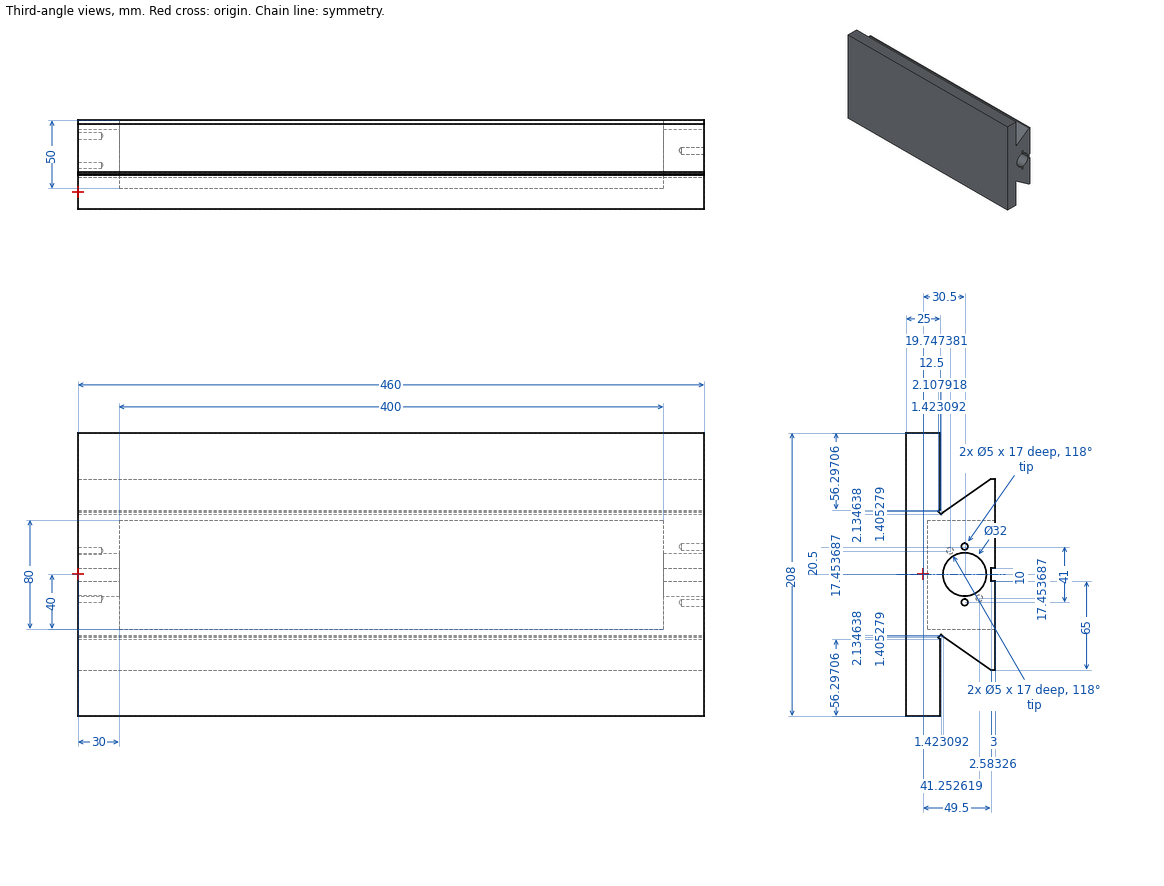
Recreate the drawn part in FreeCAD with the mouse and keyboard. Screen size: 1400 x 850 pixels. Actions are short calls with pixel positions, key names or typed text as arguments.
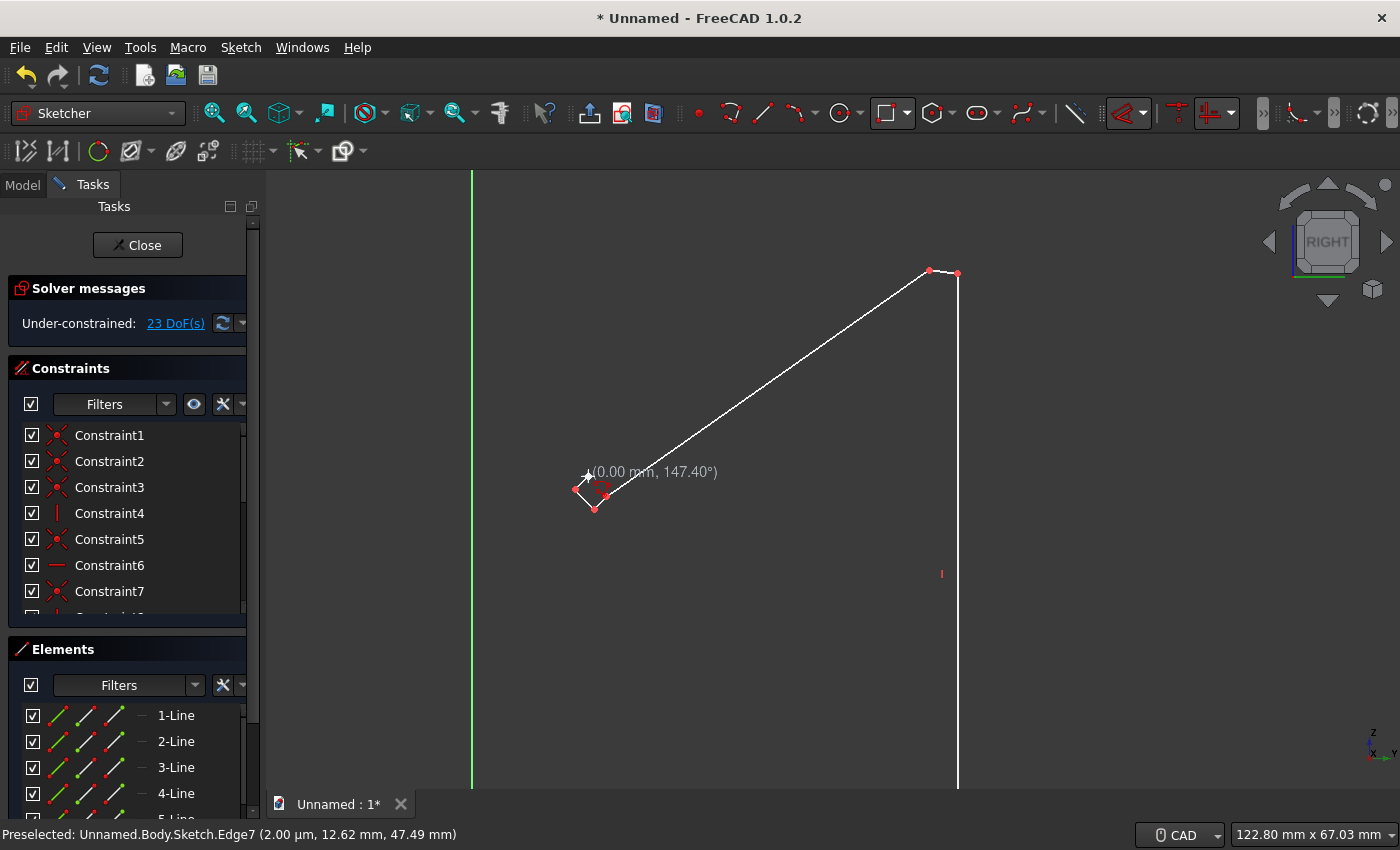
scroll(792, 369, down, 8)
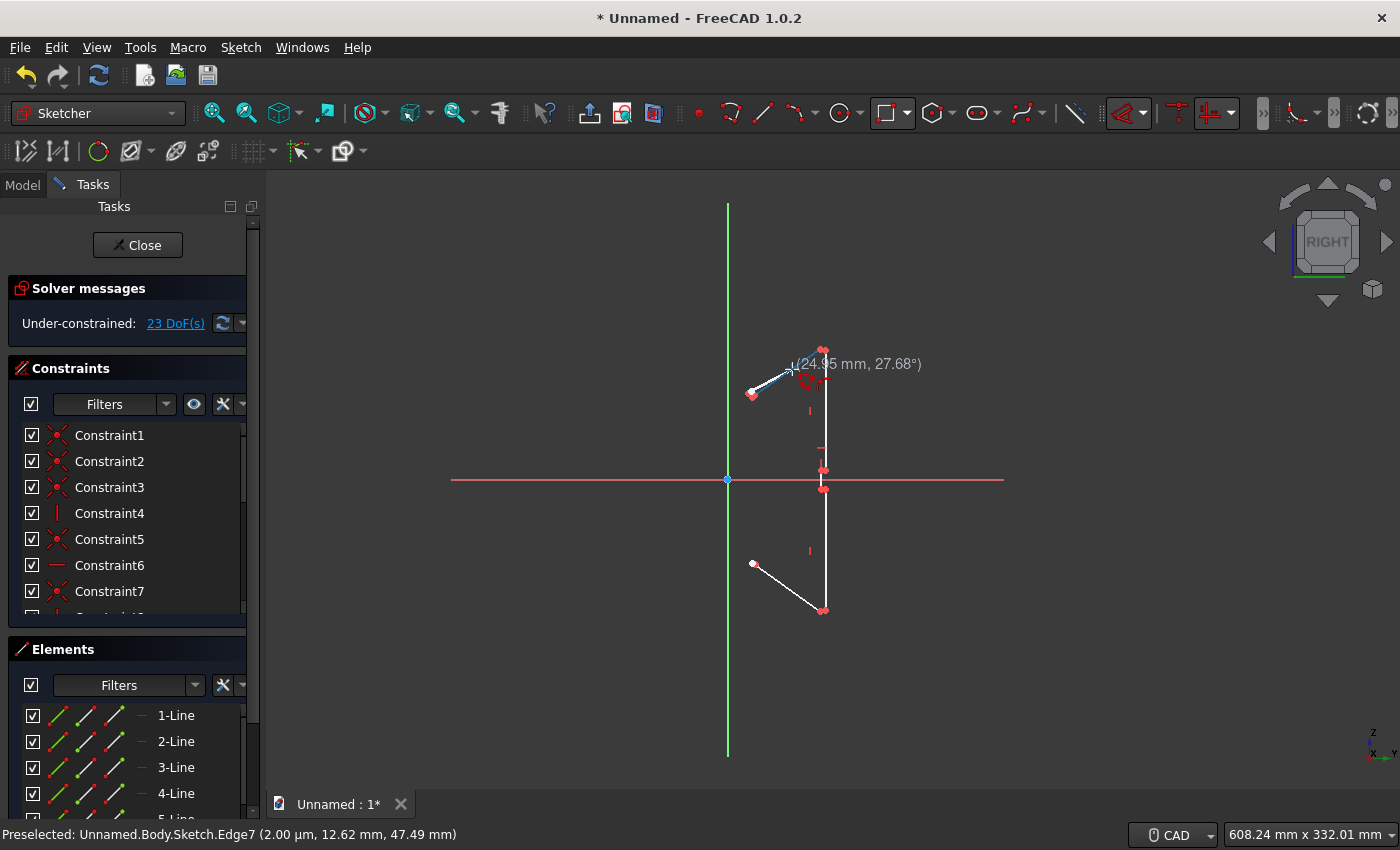
click(751, 286)
click(705, 286)
click(705, 674)
click(751, 674)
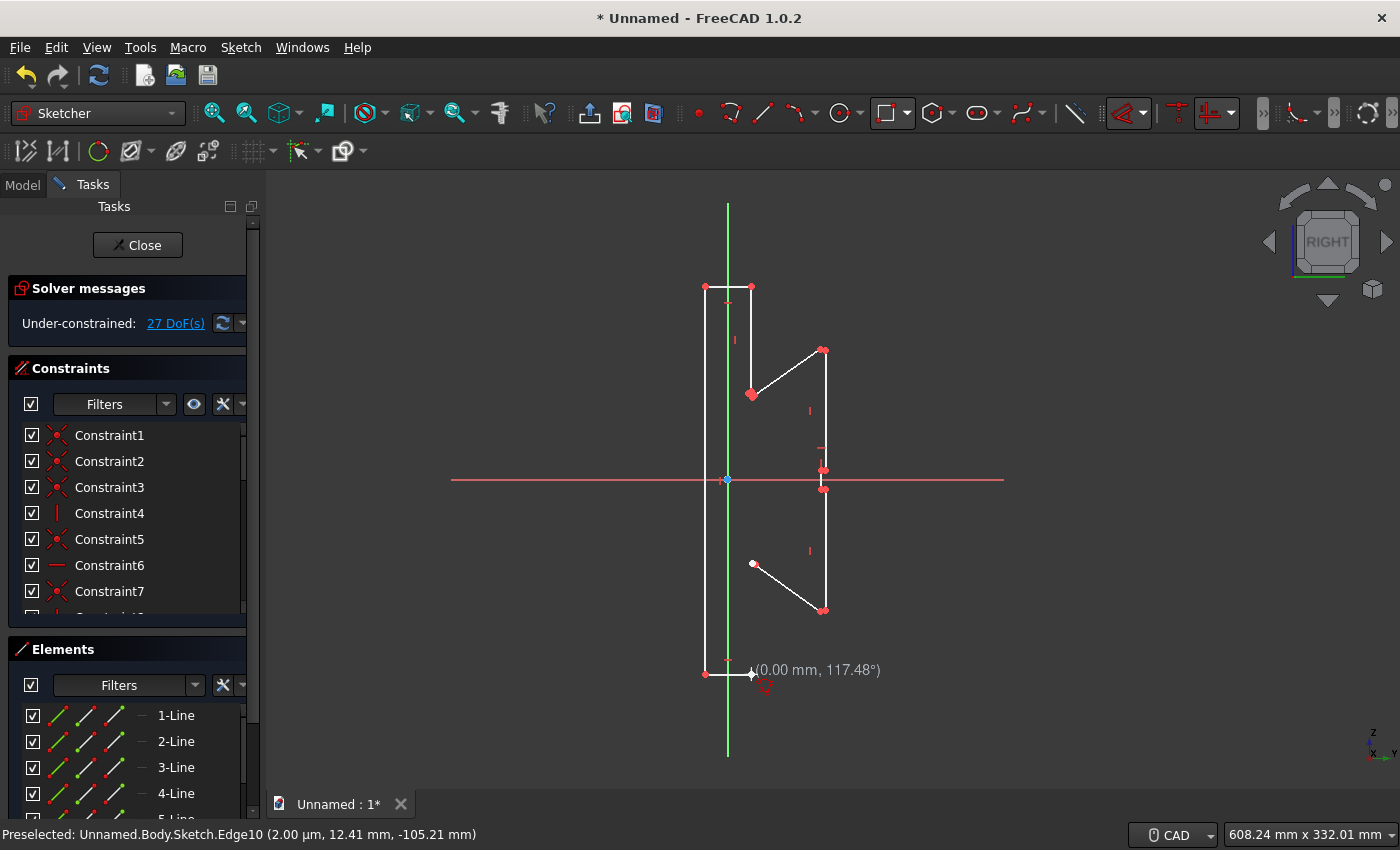
scroll(751, 569, up, 6)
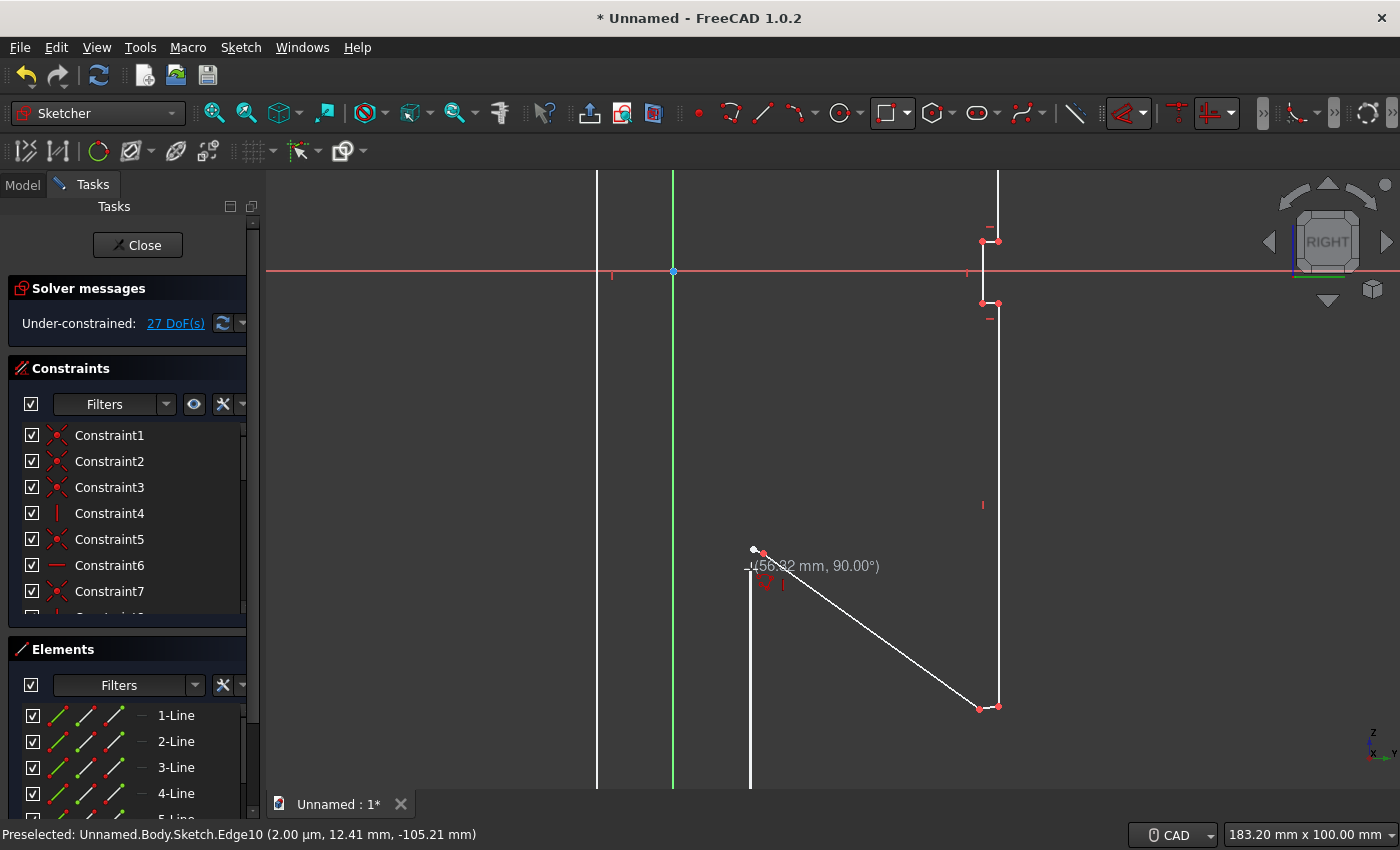
click(750, 567)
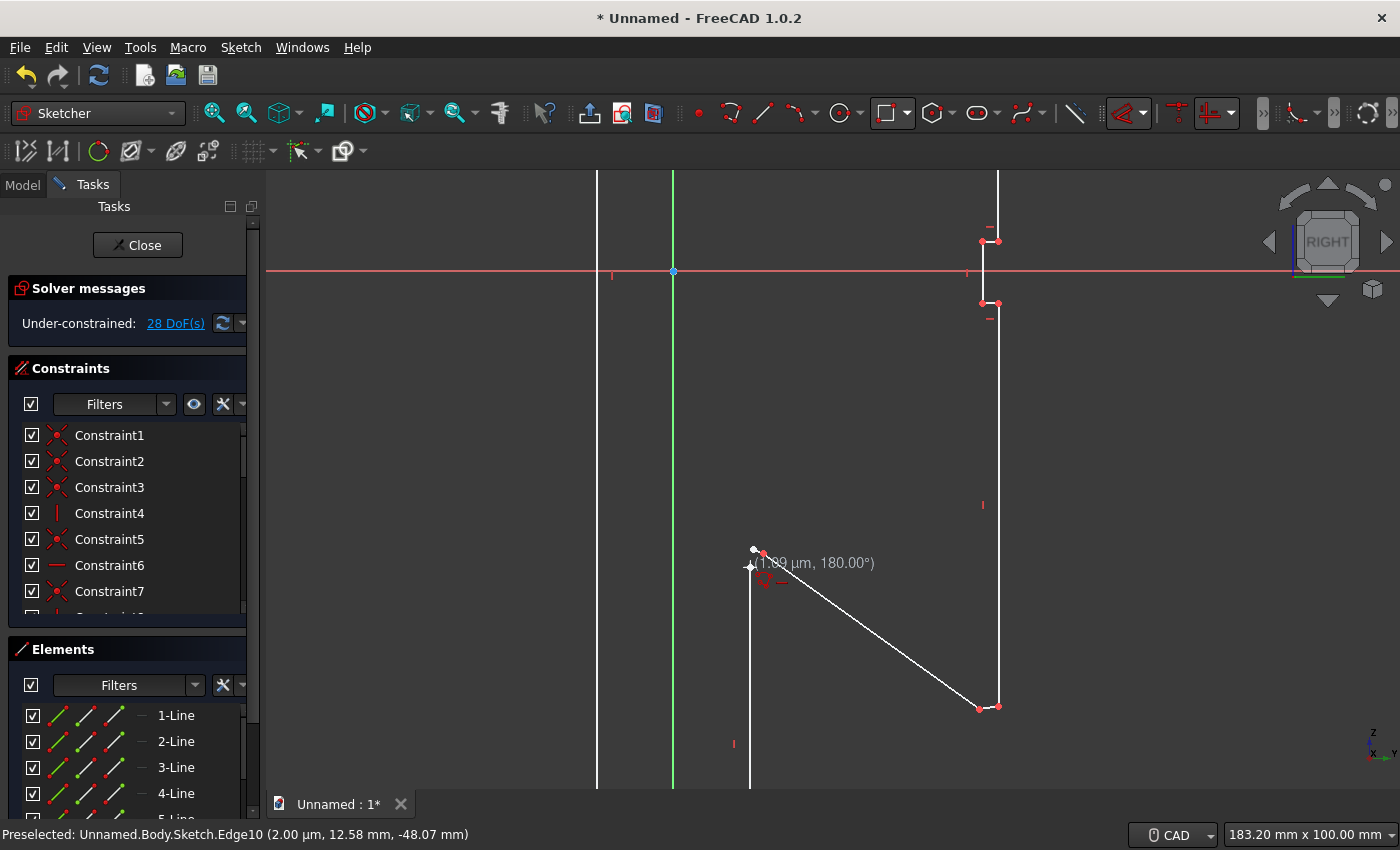
scroll(742, 558, up, 2)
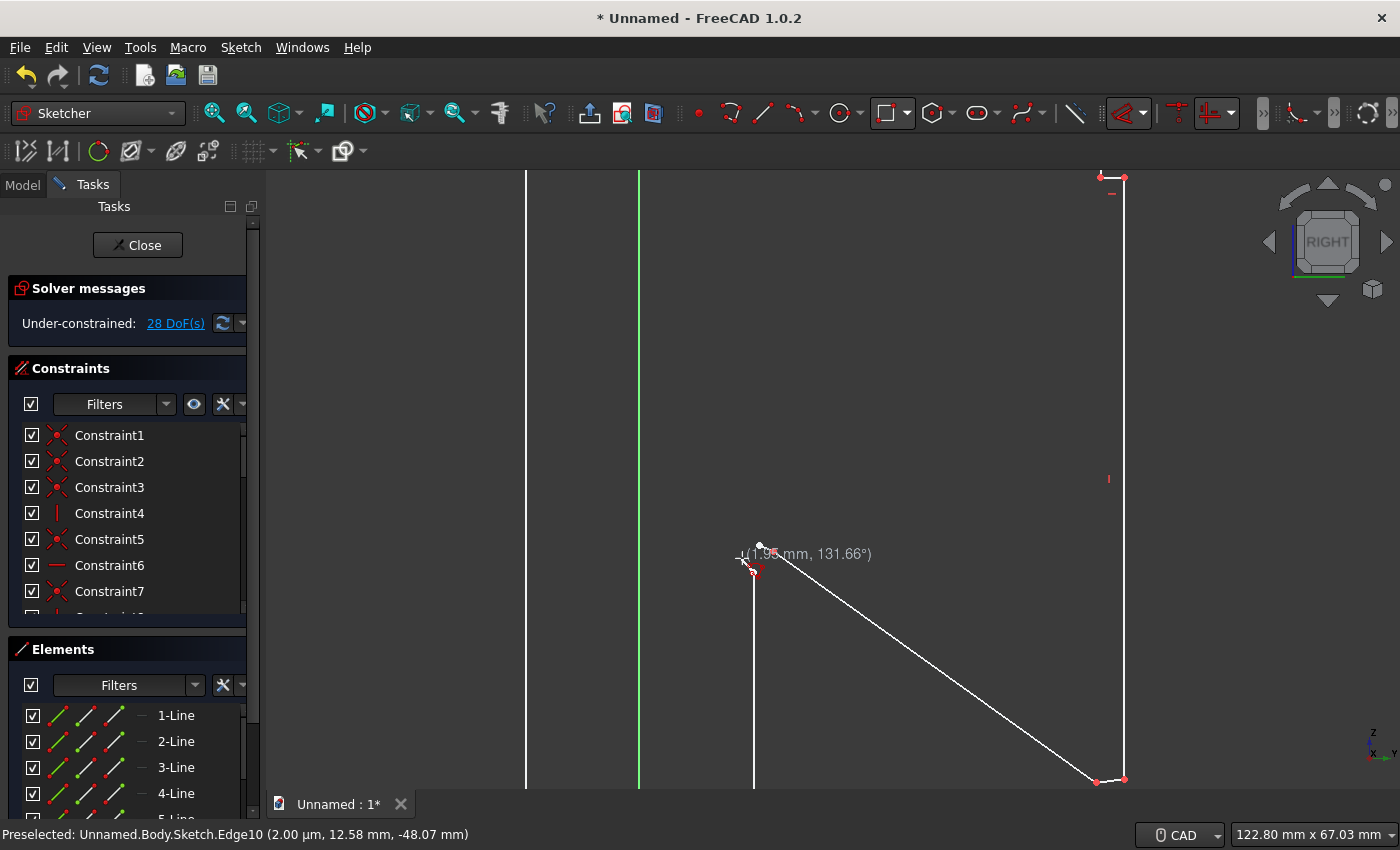
click(741, 558)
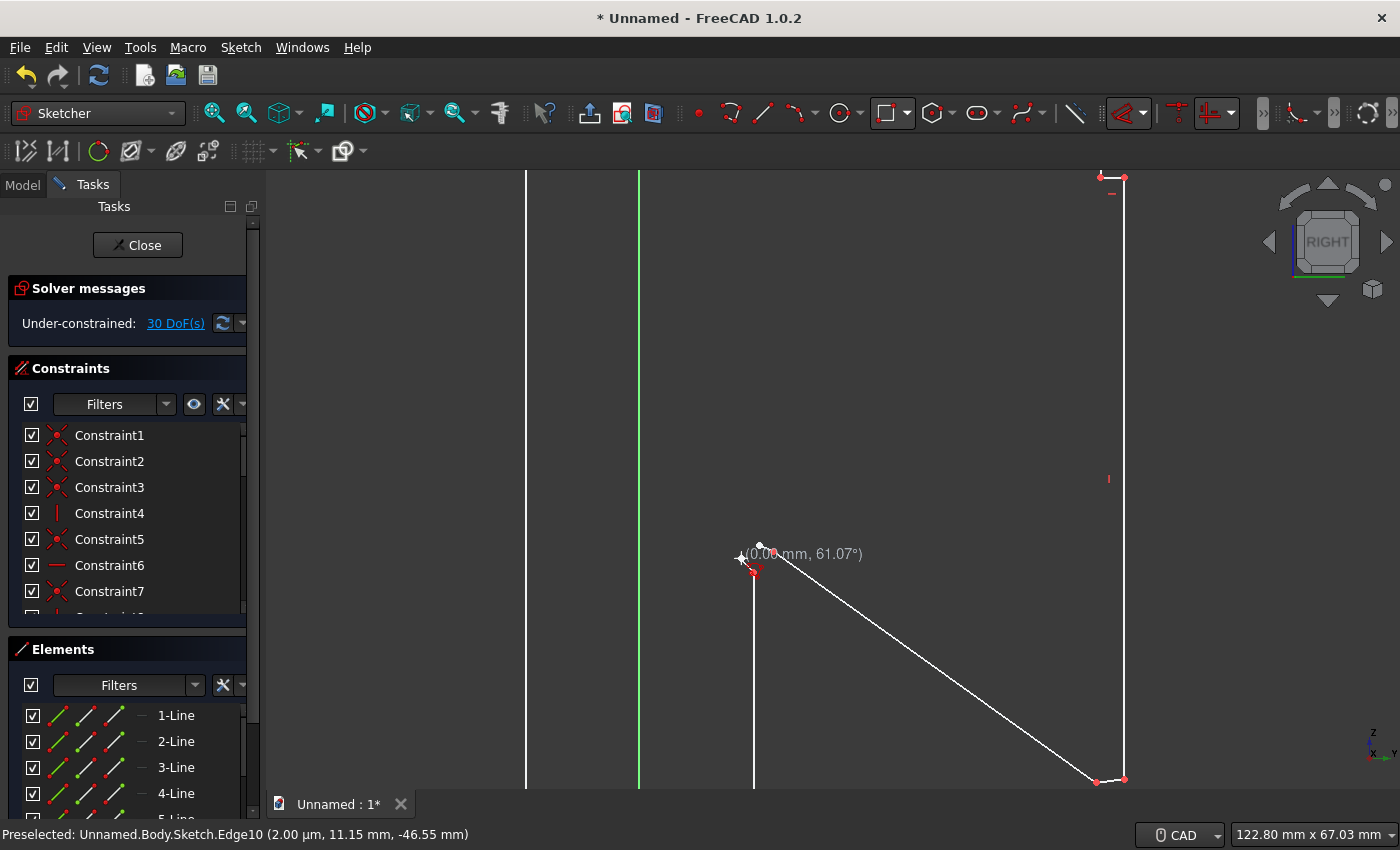
scroll(761, 538, up, 3)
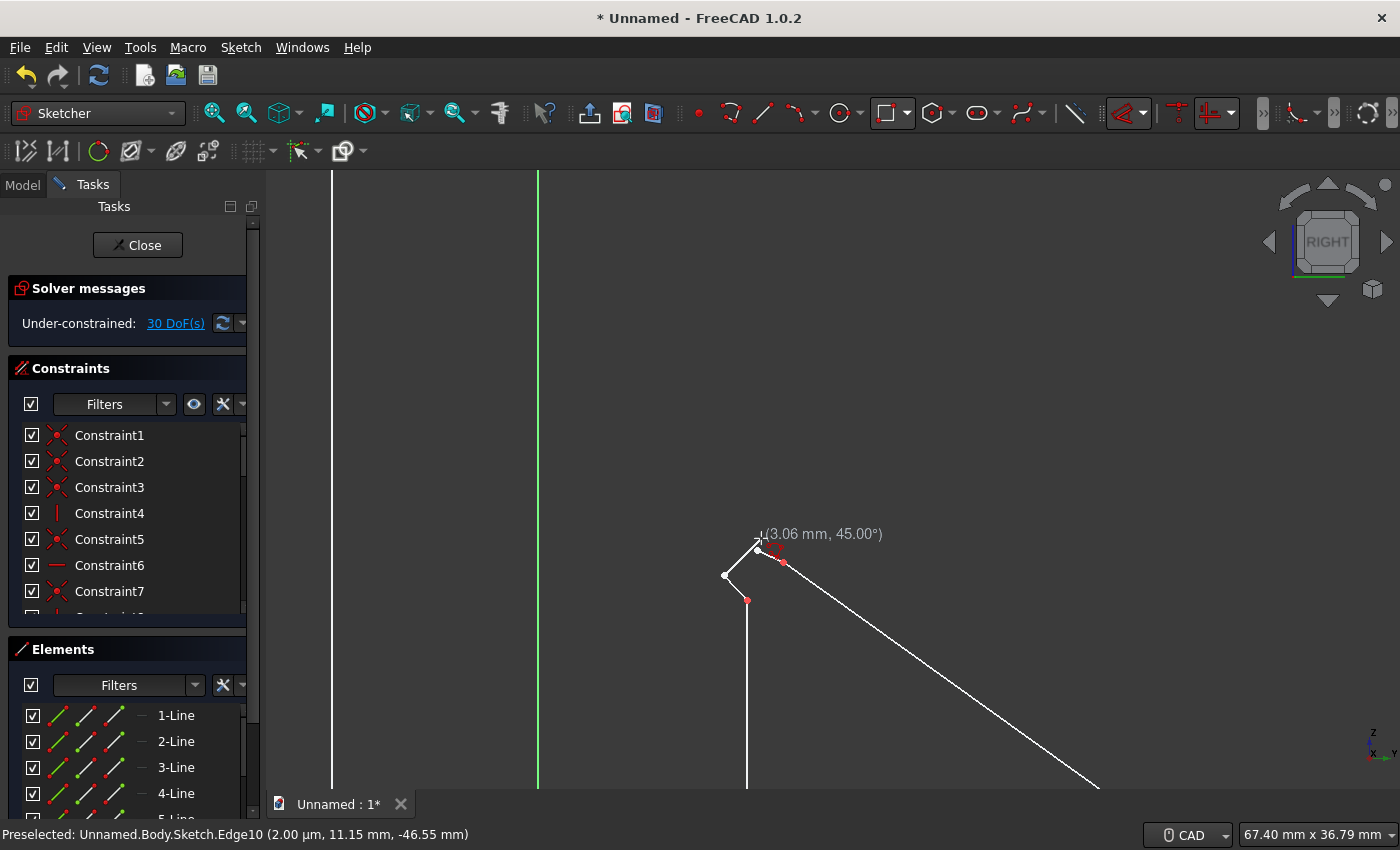
click(757, 542)
key(Escape)
key(Escape)